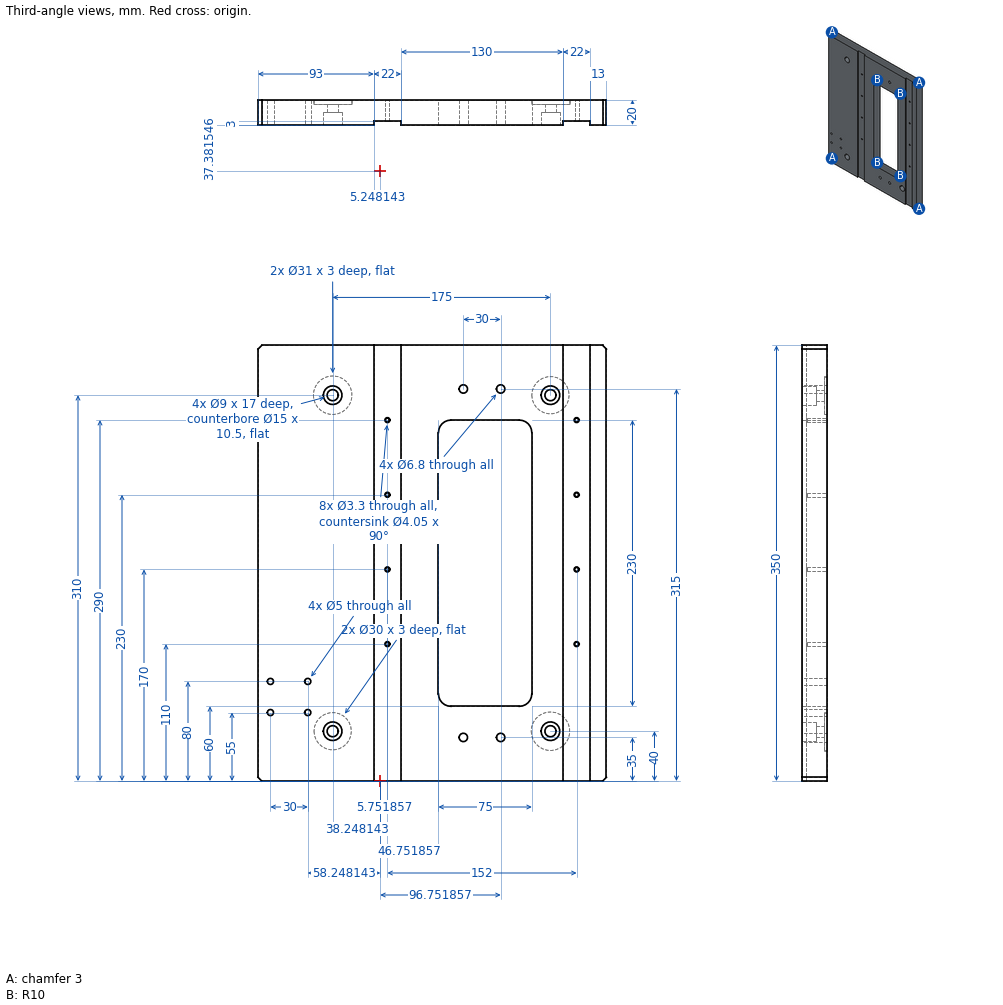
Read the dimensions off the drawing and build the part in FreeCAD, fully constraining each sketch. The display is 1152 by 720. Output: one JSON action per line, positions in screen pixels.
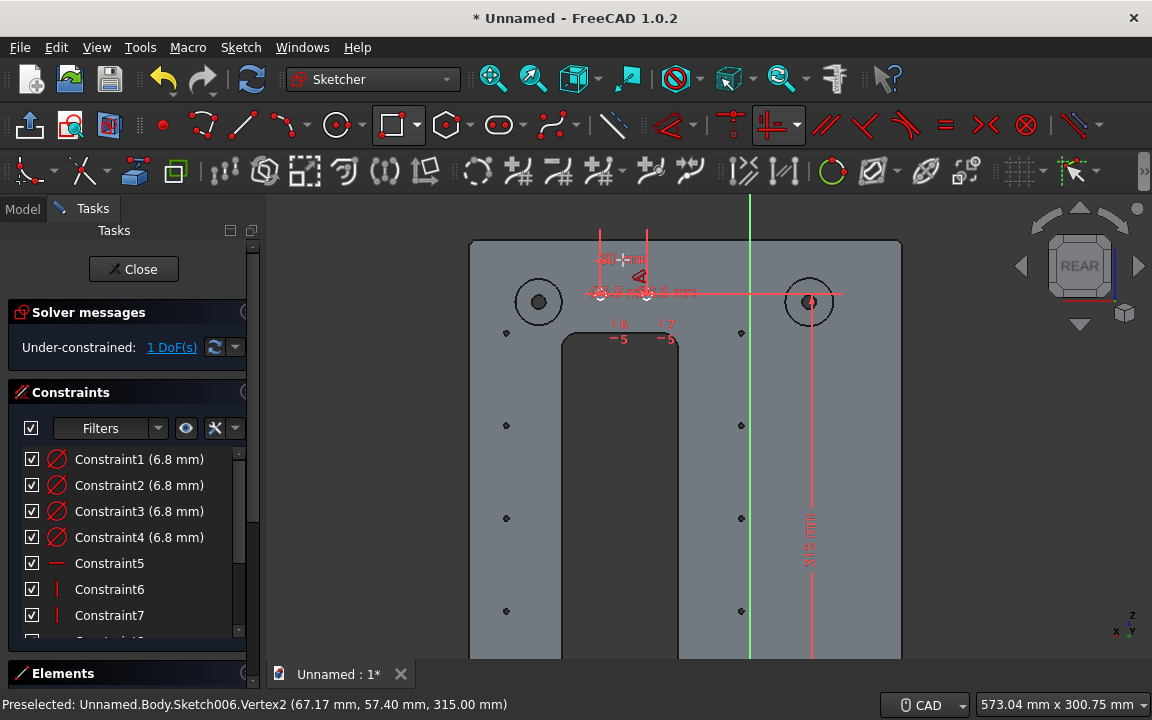
{"action": "left_click", "coordinate": [600, 294]}
{"action": "left_click", "coordinate": [710, 260]}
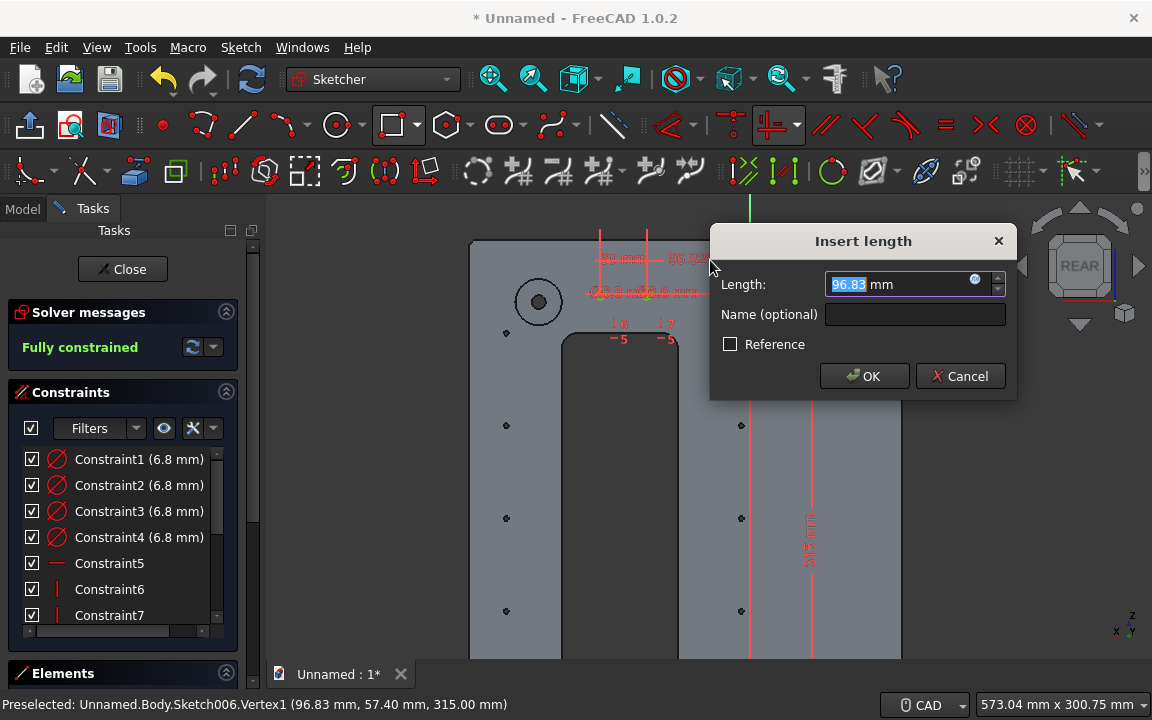
{"action": "type", "text": "96.751857"}
{"action": "key", "text": "Return"}
{"action": "key", "text": "Escape"}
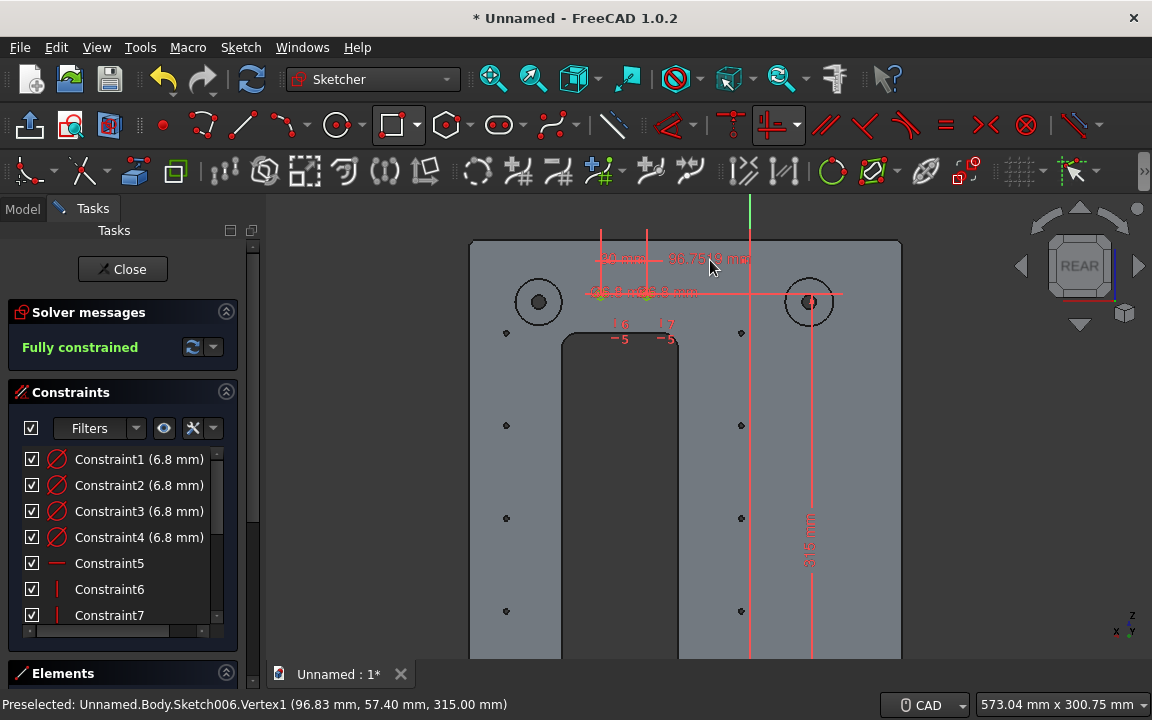
{"action": "left_click", "coordinate": [123, 269]}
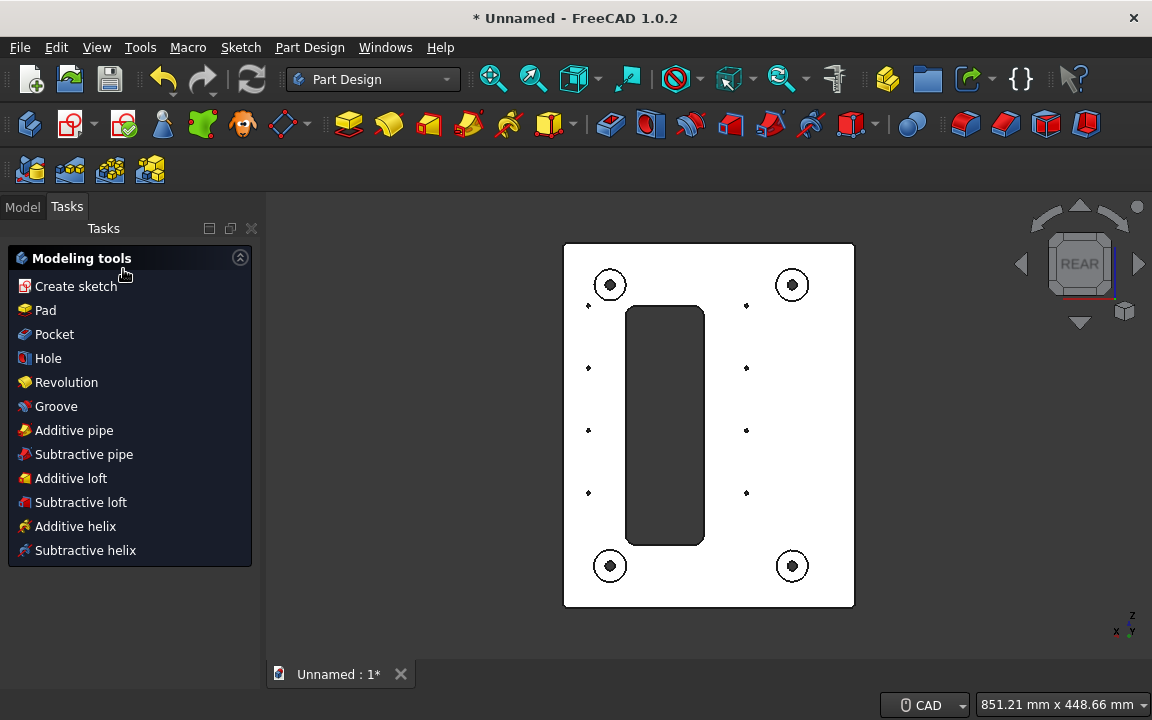
{"action": "left_click", "coordinate": [652, 124]}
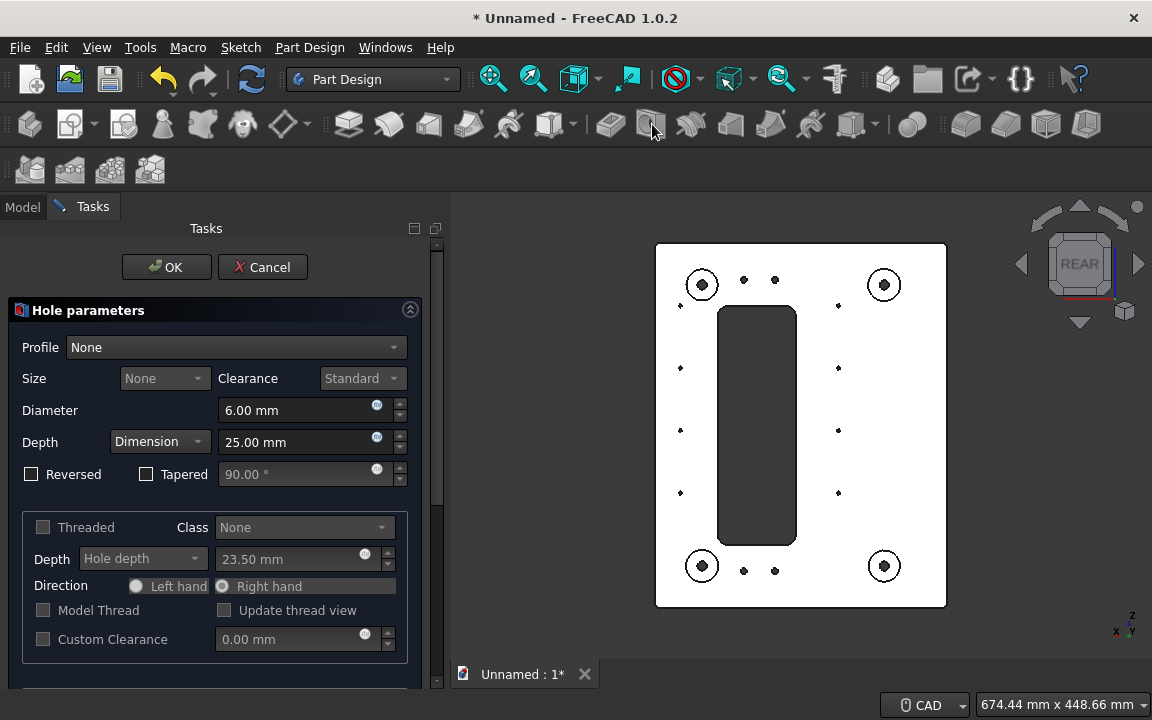
{"action": "triple_click", "coordinate": [305, 410]}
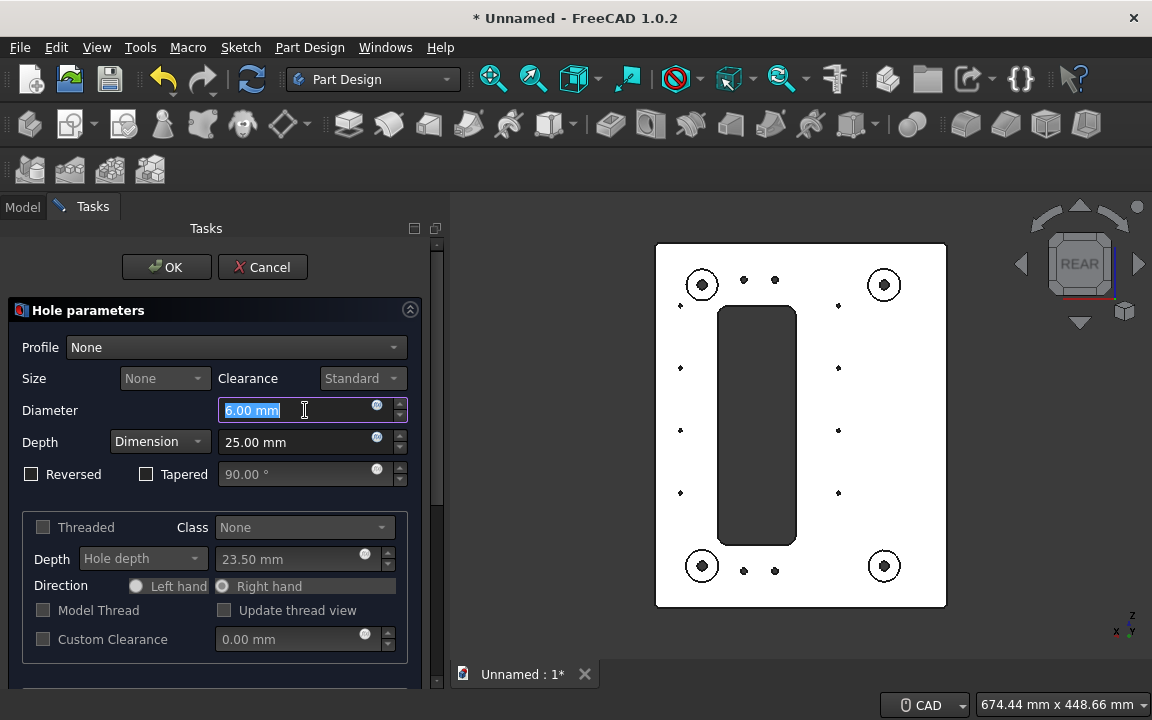
{"action": "type", "text": "6.8"}
{"action": "key", "text": "Tab"}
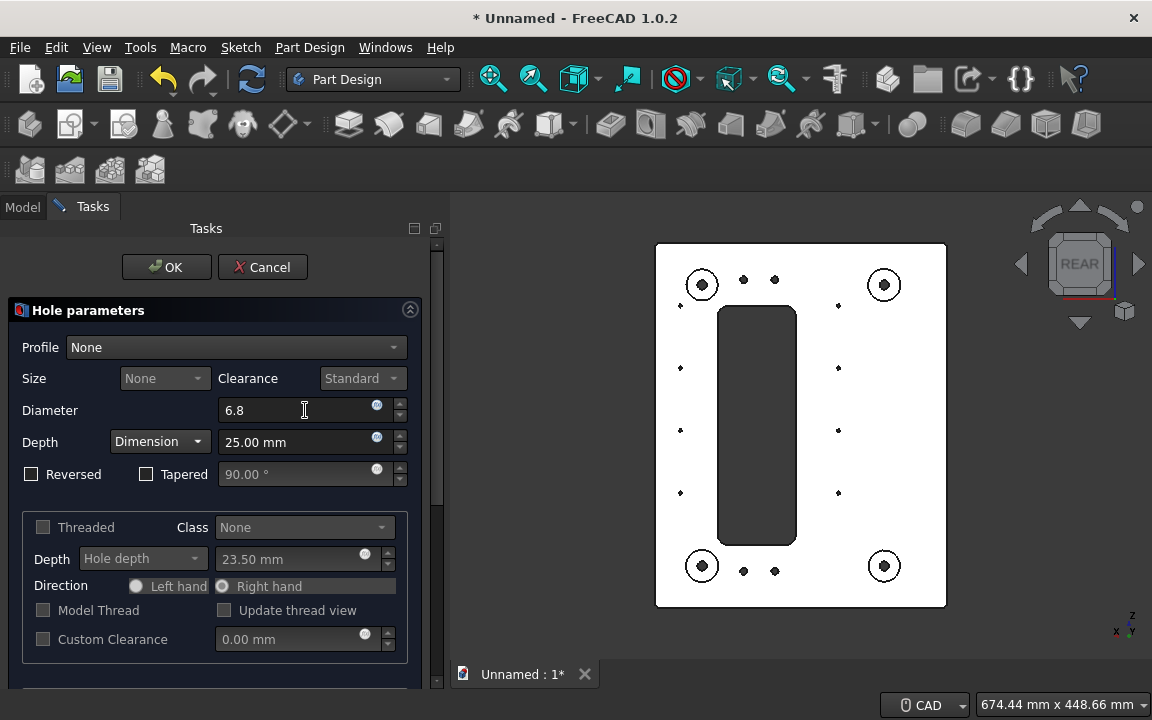
{"action": "left_click", "coordinate": [161, 442]}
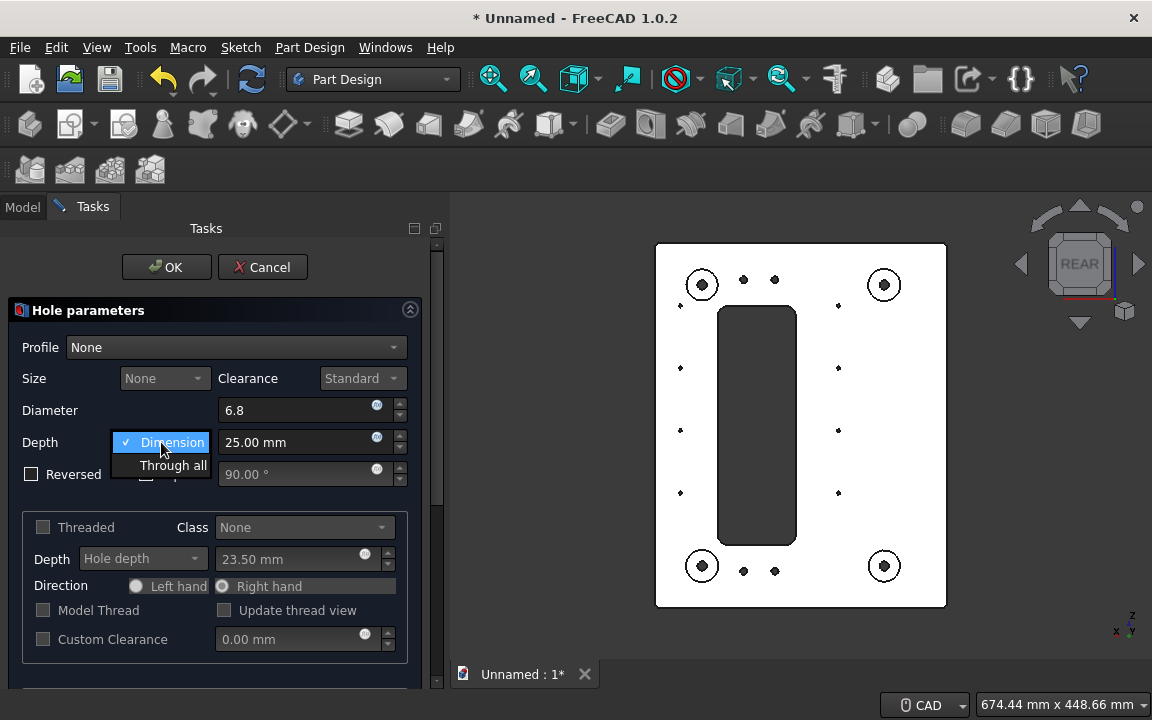
{"action": "left_click", "coordinate": [160, 466]}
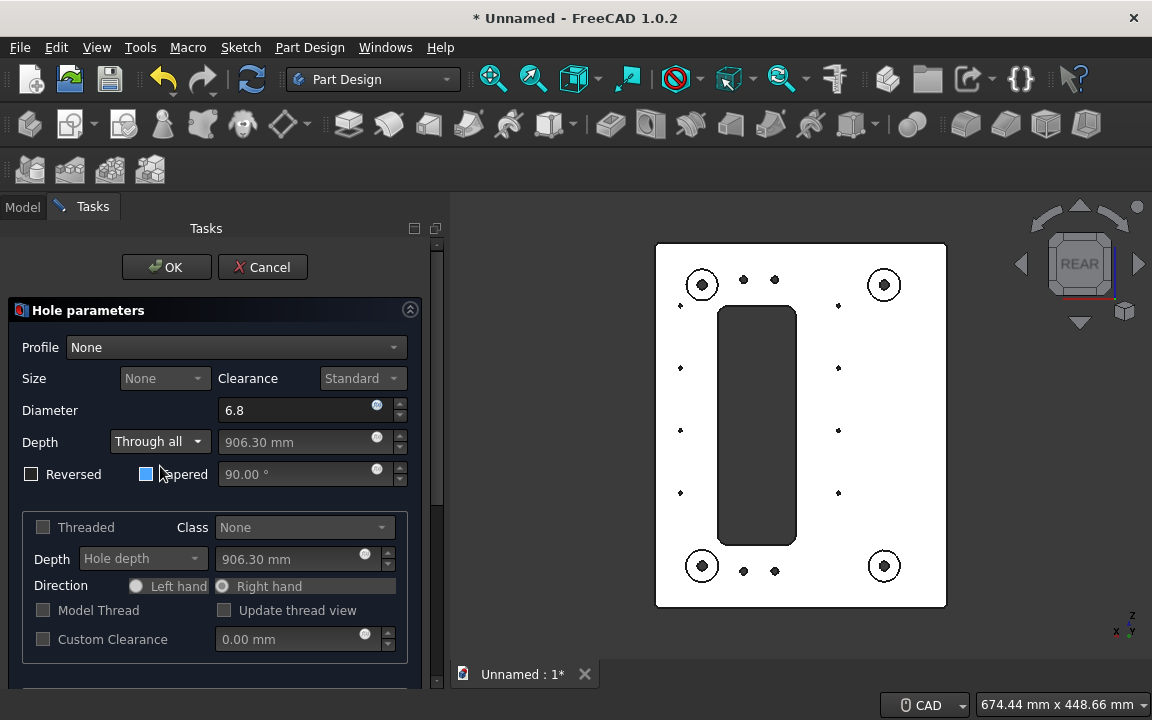
{"action": "left_click", "coordinate": [167, 267]}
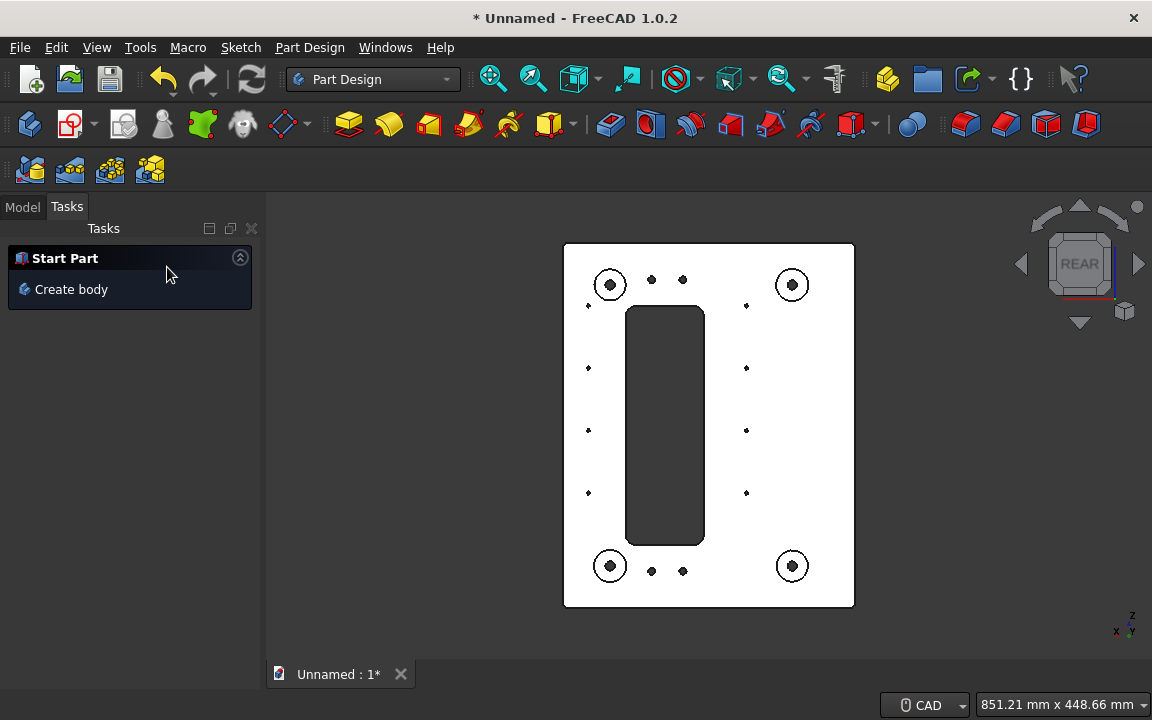
{"action": "left_click", "coordinate": [792, 477]}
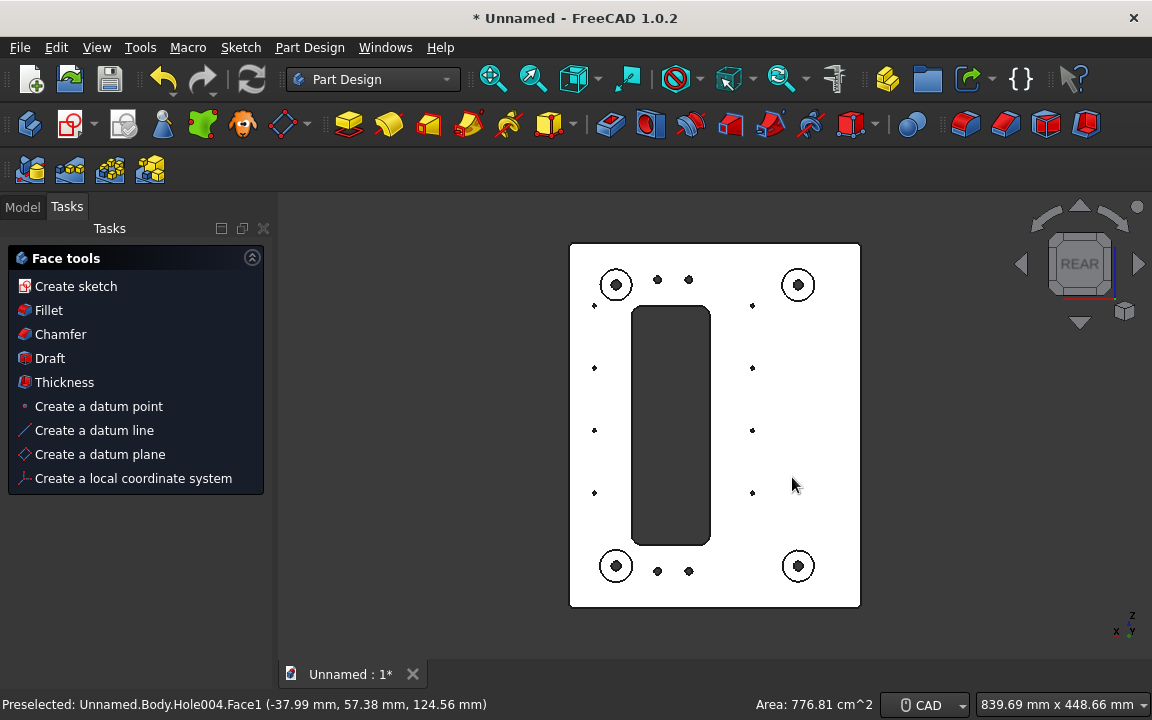
{"action": "left_click", "coordinate": [70, 124]}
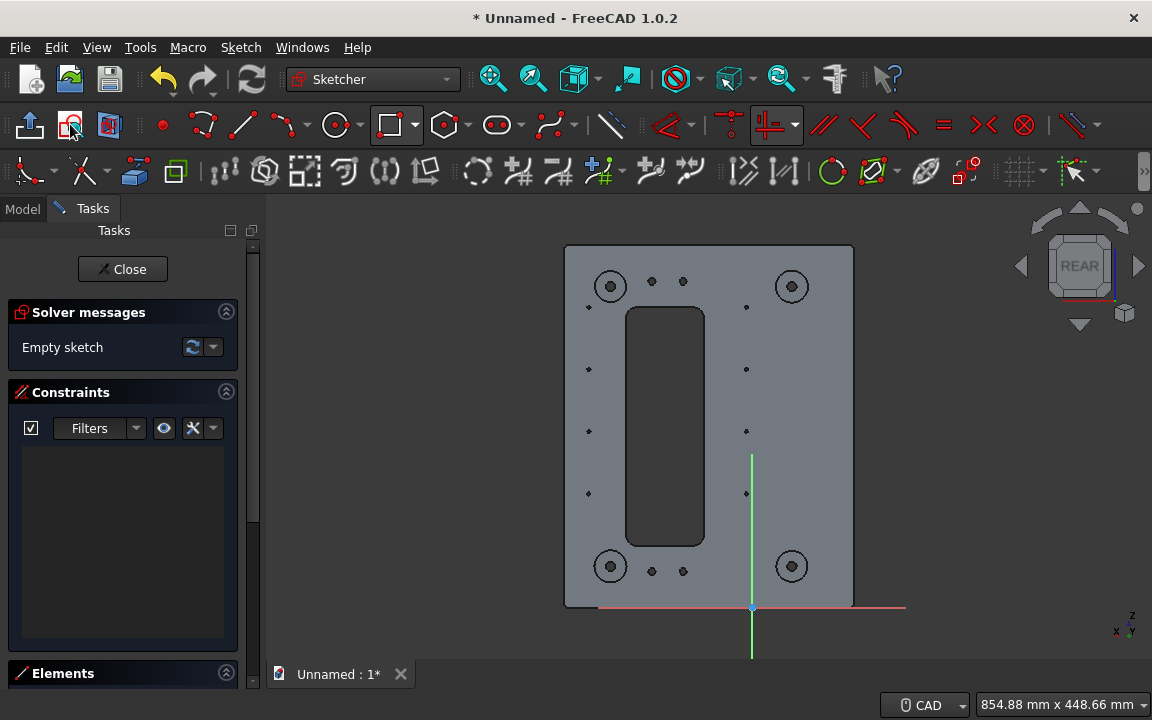
{"action": "scroll", "coordinate": [852, 552], "scroll_direction": "up", "scroll_amount": 11}